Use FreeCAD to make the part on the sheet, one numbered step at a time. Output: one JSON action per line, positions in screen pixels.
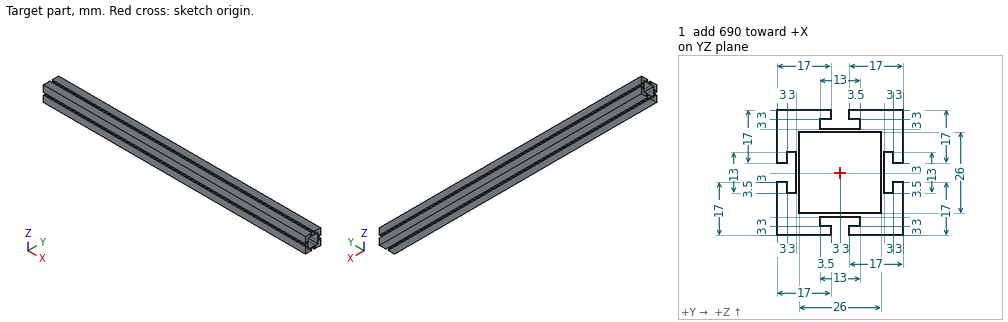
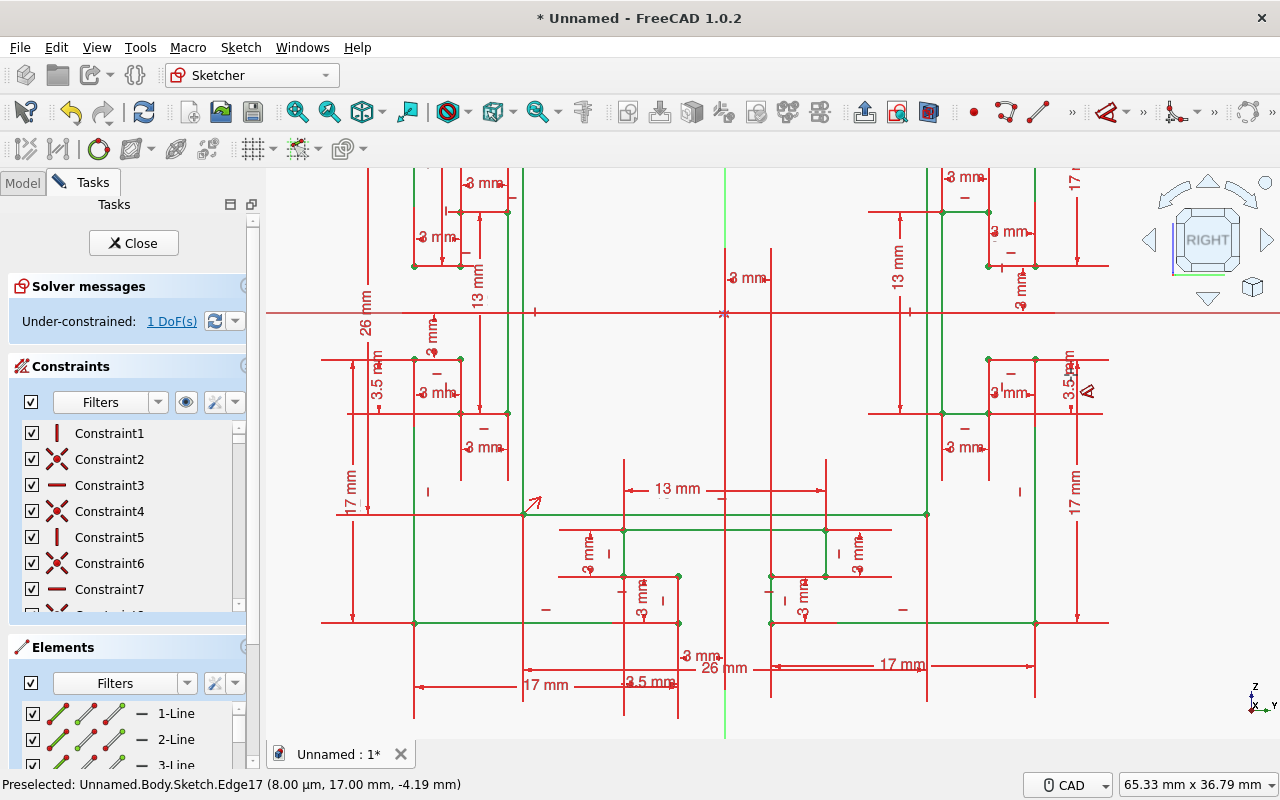
{"action": "scroll", "coordinate": [680, 624], "scroll_direction": "down", "scroll_amount": 3}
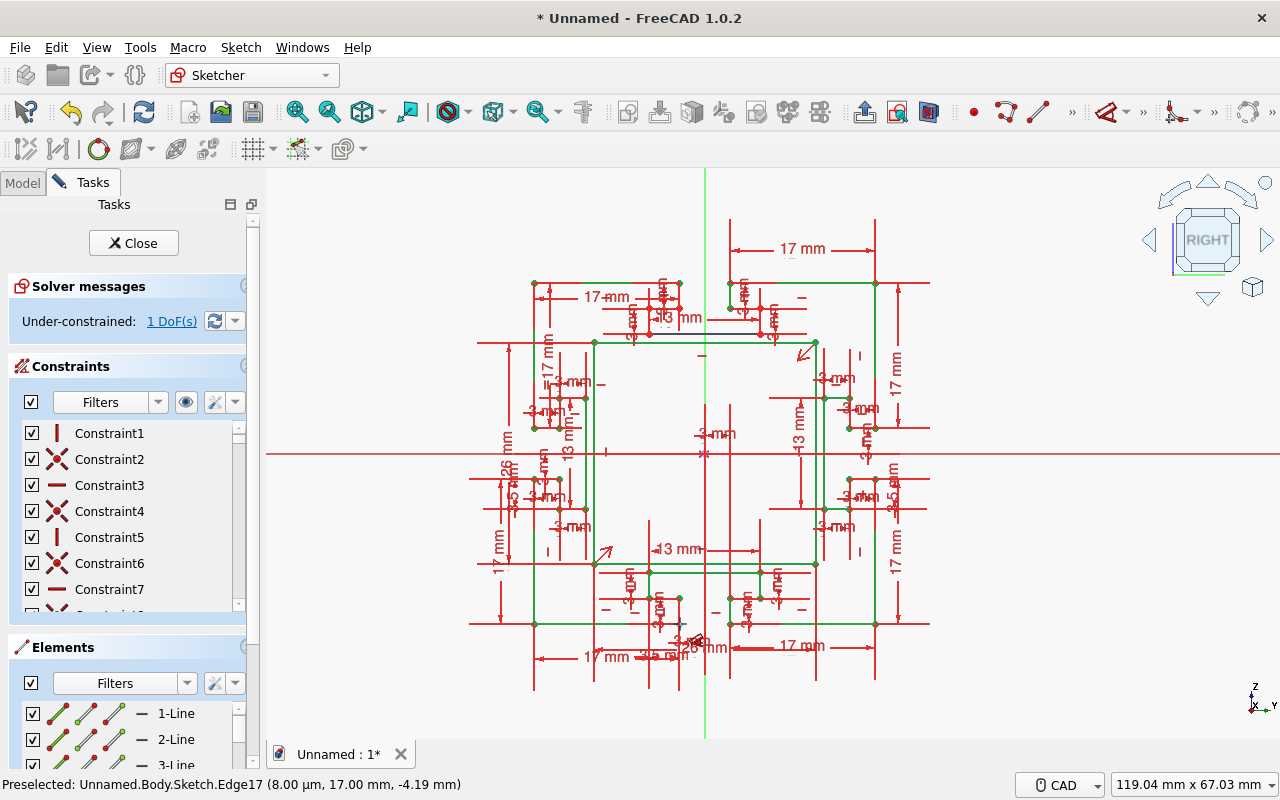
{"action": "scroll", "coordinate": [739, 309], "scroll_direction": "up", "scroll_amount": 3}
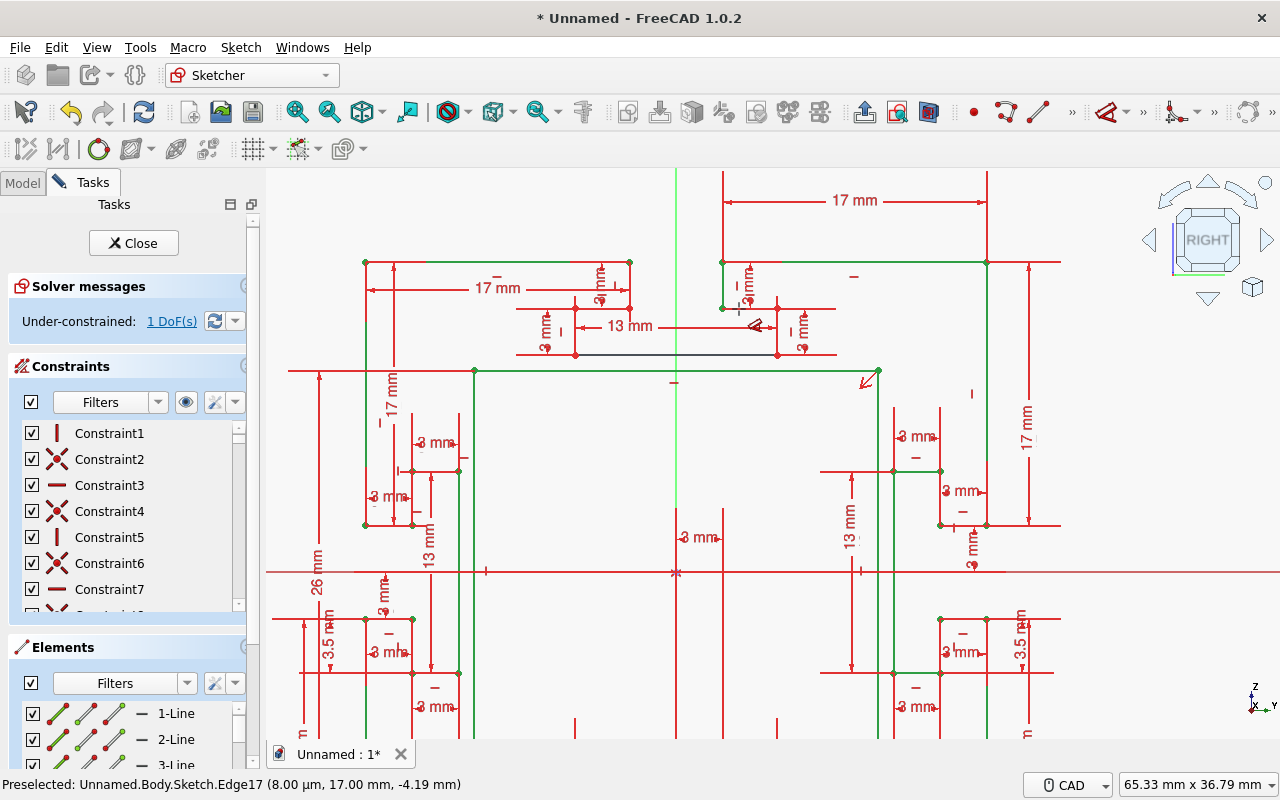
{"action": "left_click", "coordinate": [739, 309]}
{"action": "left_click", "coordinate": [750, 227]}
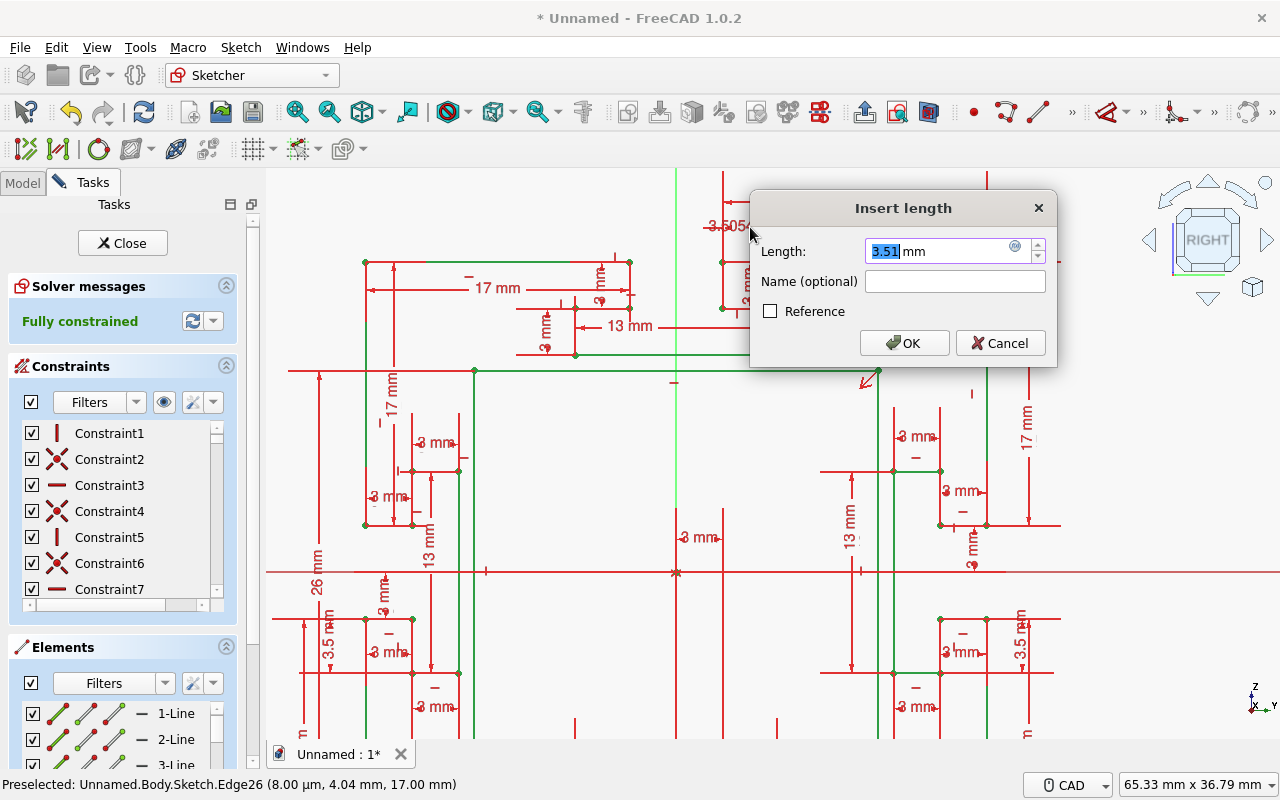
{"action": "type", "text": "3.5"}
{"action": "key", "text": "Return"}
{"action": "key", "text": "Escape"}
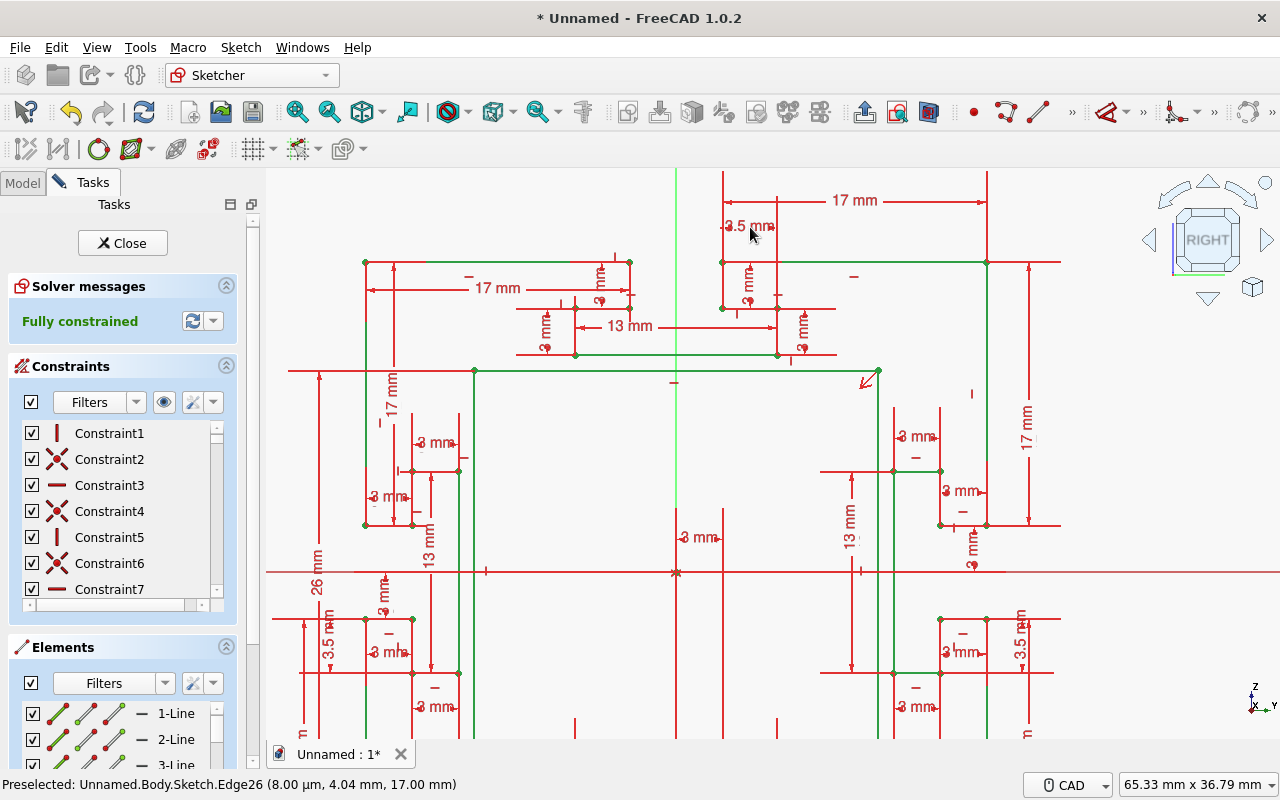
{"action": "left_click", "coordinate": [123, 243]}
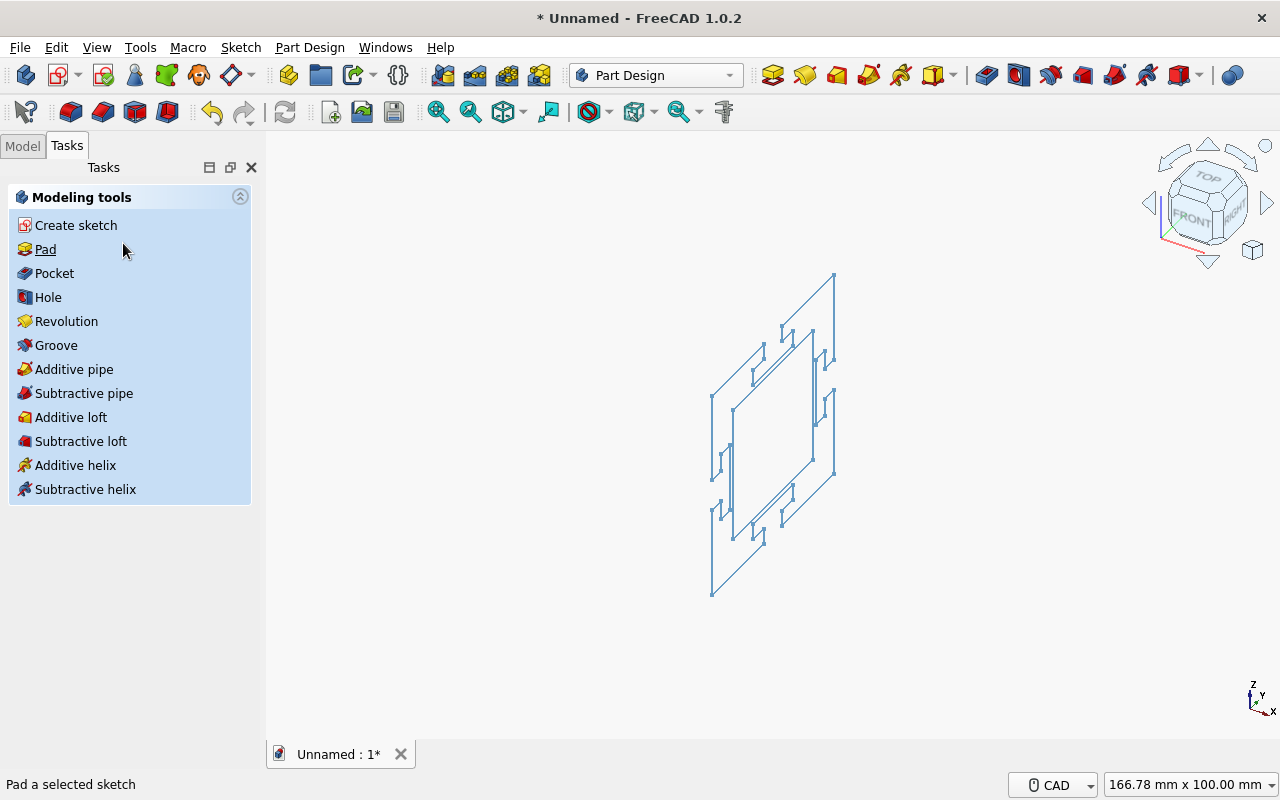
{"action": "left_click", "coordinate": [774, 76]}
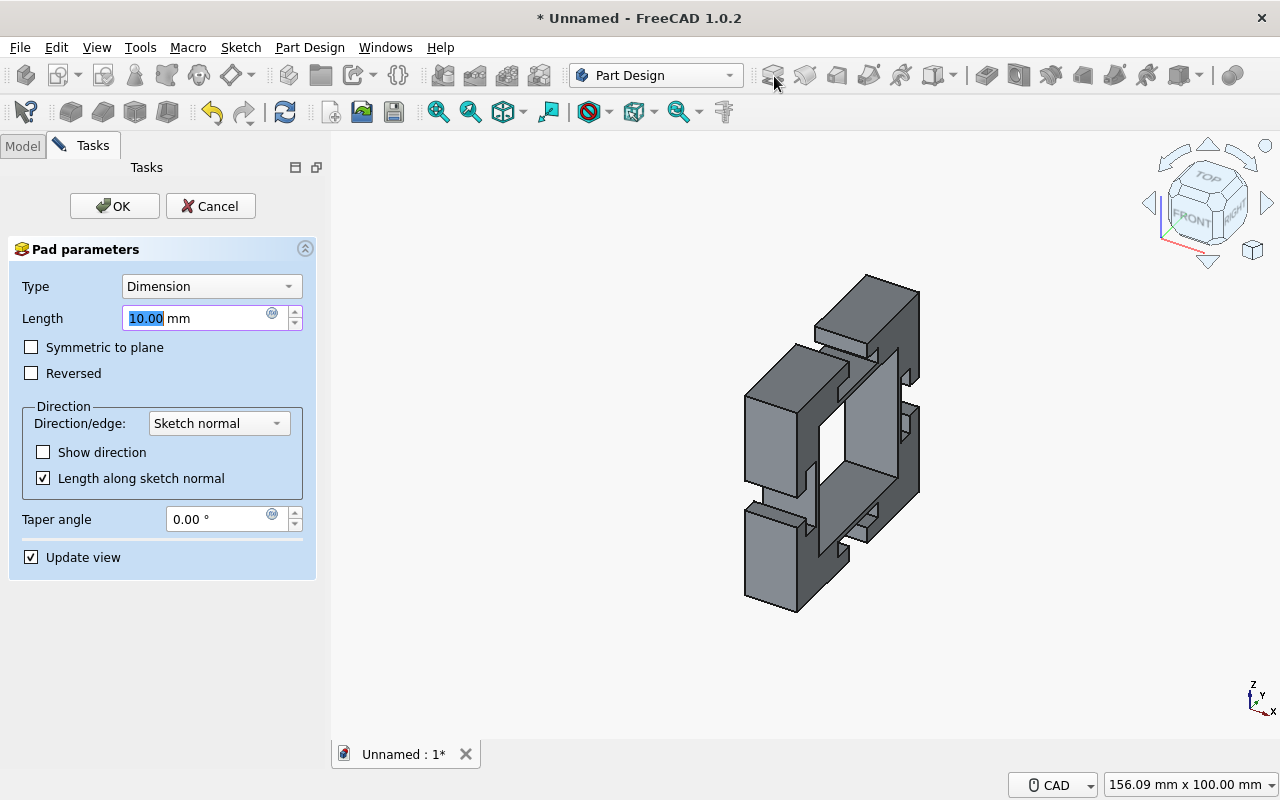
{"action": "type", "text": "690"}
{"action": "key", "text": "Tab"}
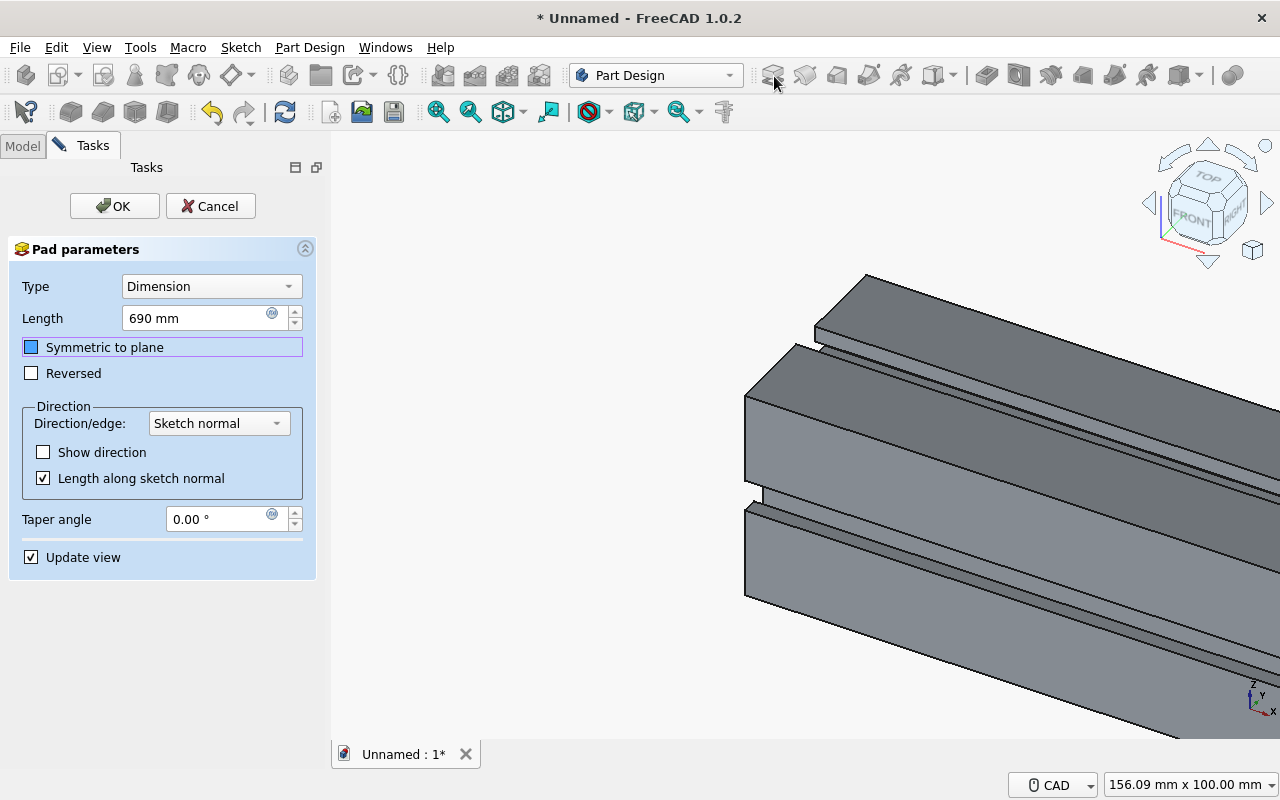
{"action": "left_click", "coordinate": [115, 206]}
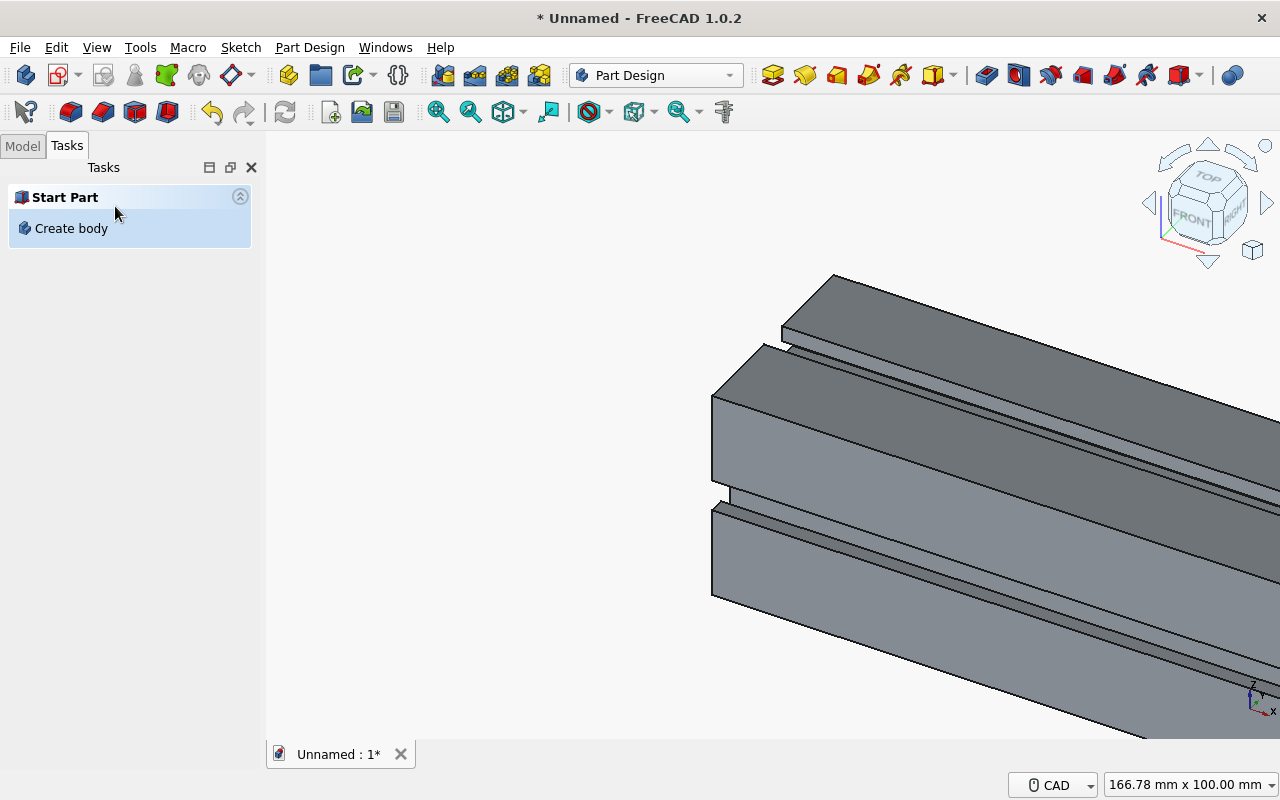
{"action": "key", "text": "0"}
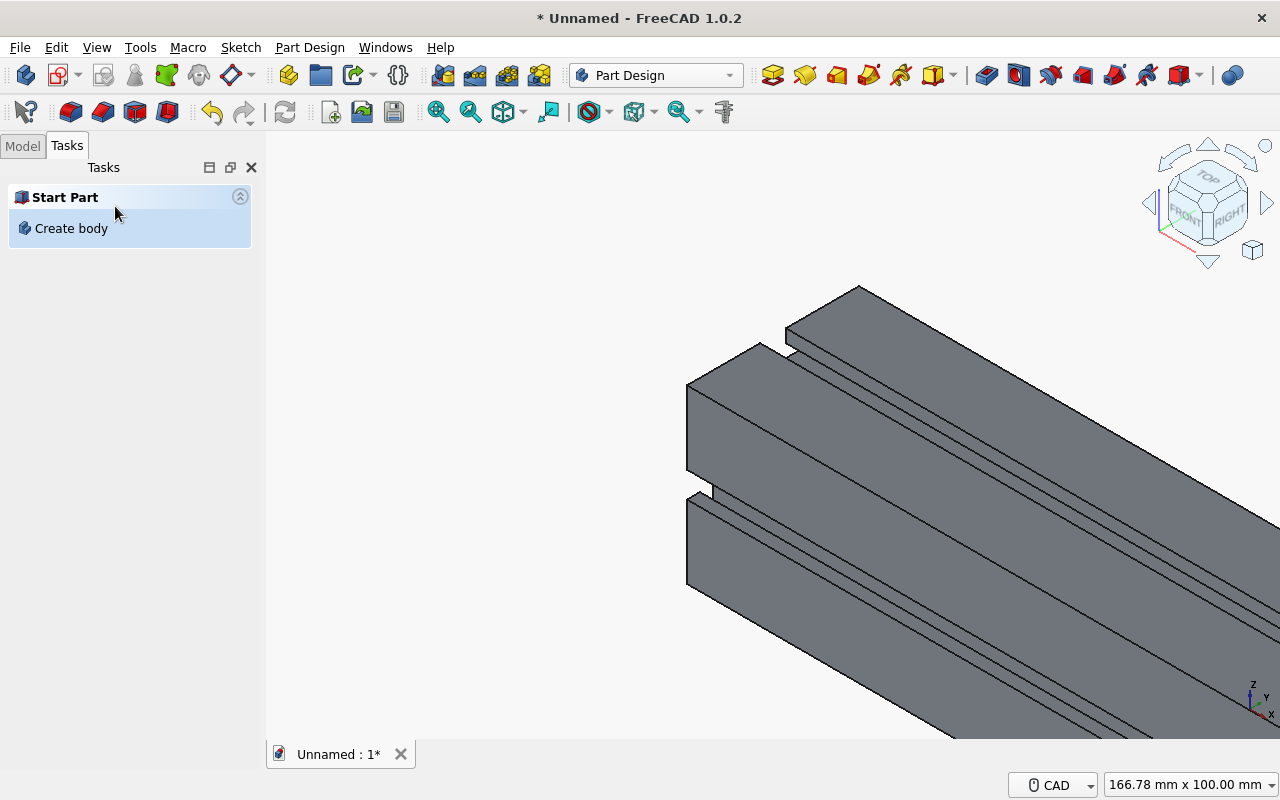
{"action": "key", "text": "v f"}